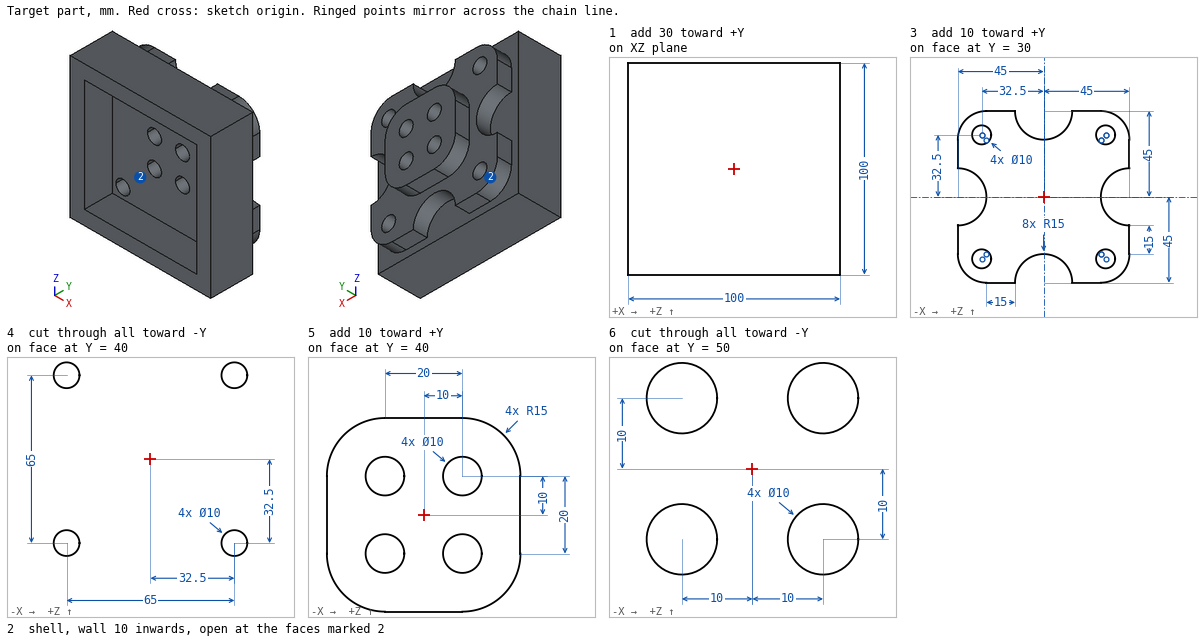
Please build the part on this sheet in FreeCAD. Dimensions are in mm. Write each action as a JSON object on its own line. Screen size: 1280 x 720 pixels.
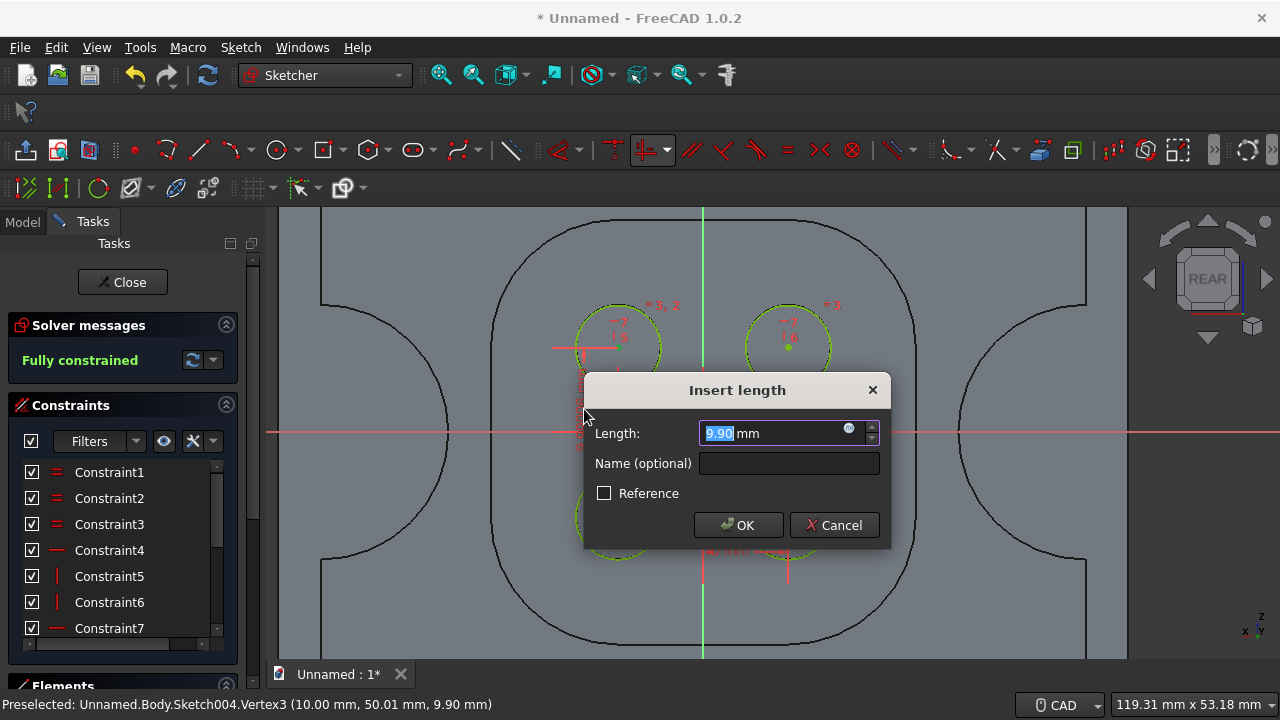
{"action": "type", "text": "10"}
{"action": "key", "text": "Return"}
{"action": "key", "text": "Escape"}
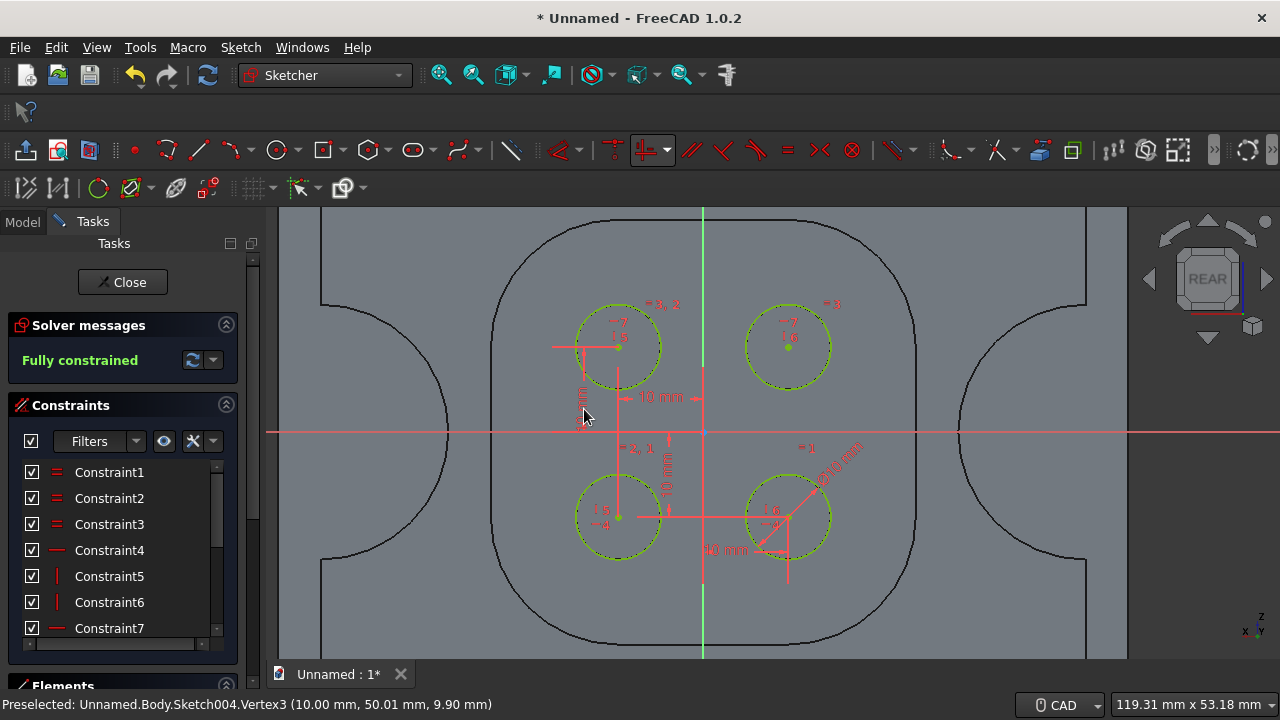
{"action": "left_click", "coordinate": [123, 282]}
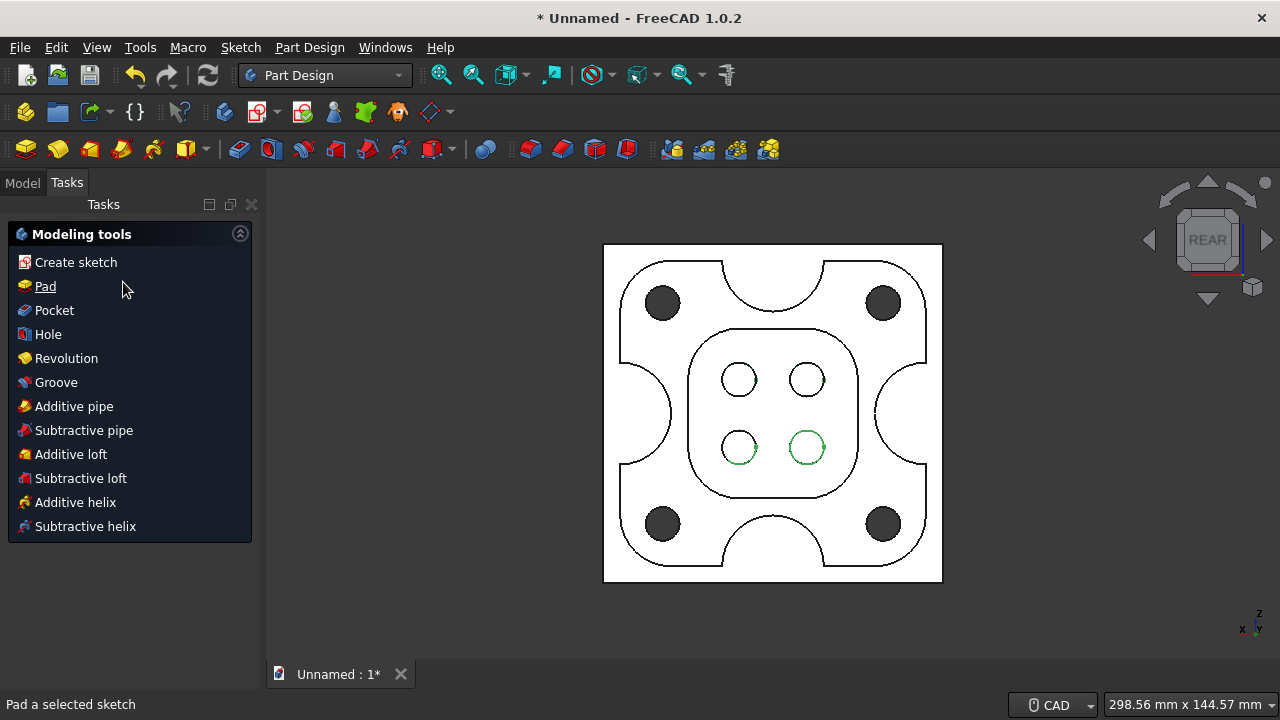
{"action": "left_click", "coordinate": [240, 150]}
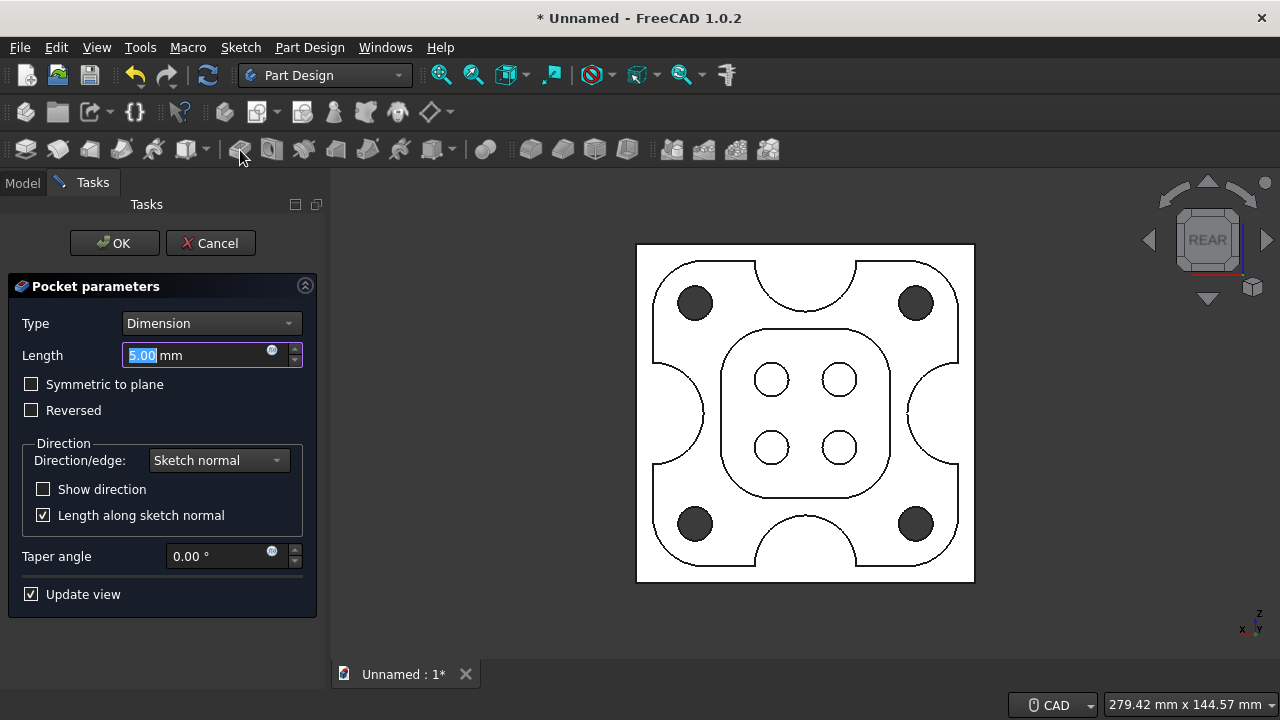
{"action": "left_click", "coordinate": [212, 324]}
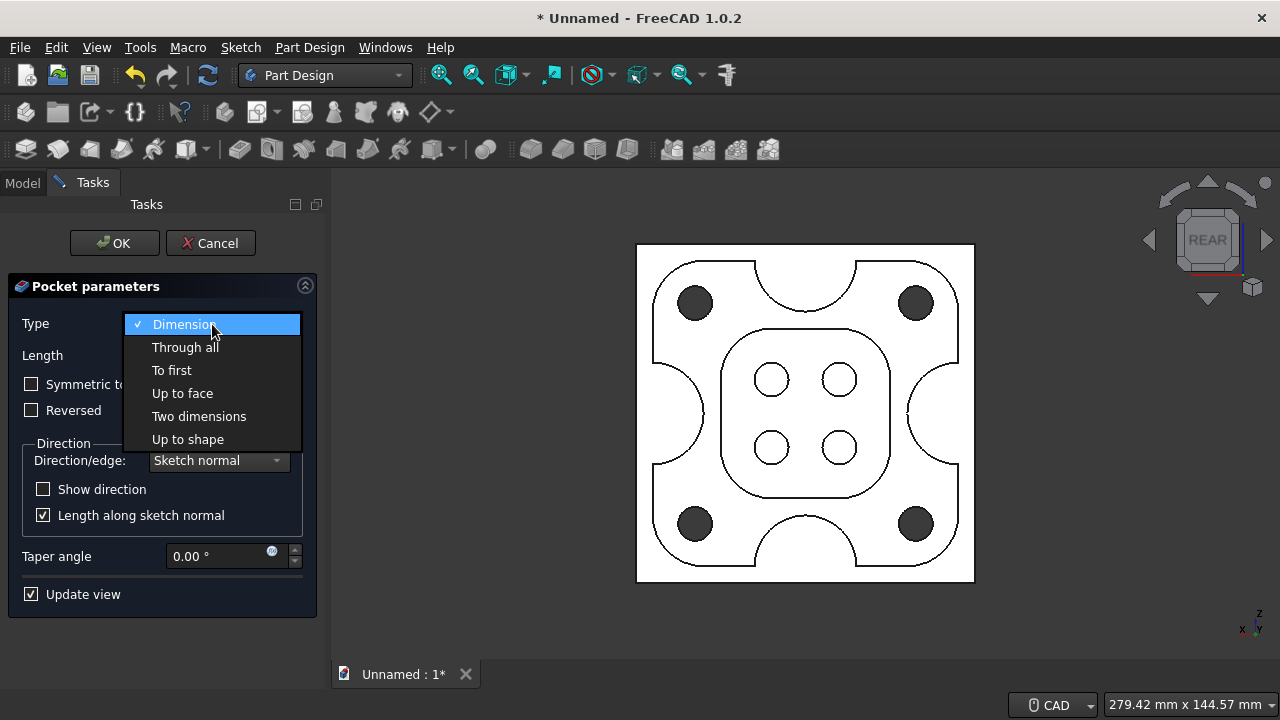
{"action": "left_click", "coordinate": [212, 348]}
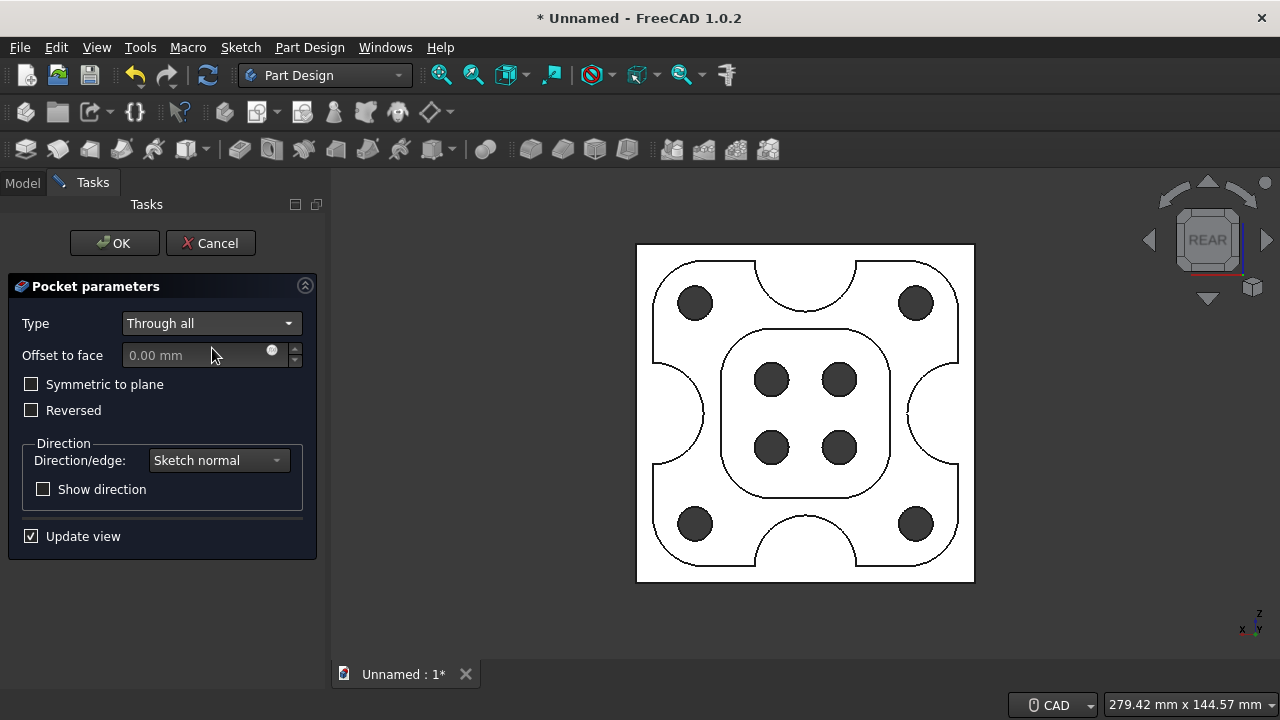
{"action": "left_click", "coordinate": [115, 243]}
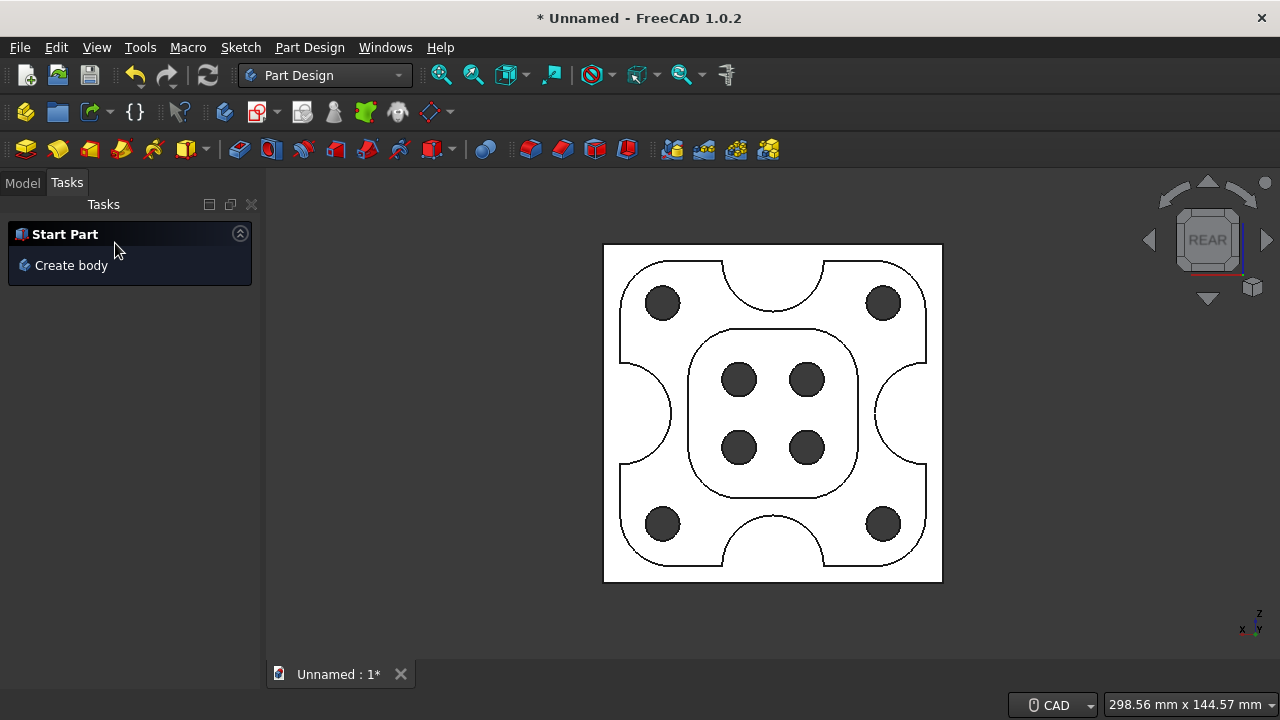
{"action": "key", "text": "0"}